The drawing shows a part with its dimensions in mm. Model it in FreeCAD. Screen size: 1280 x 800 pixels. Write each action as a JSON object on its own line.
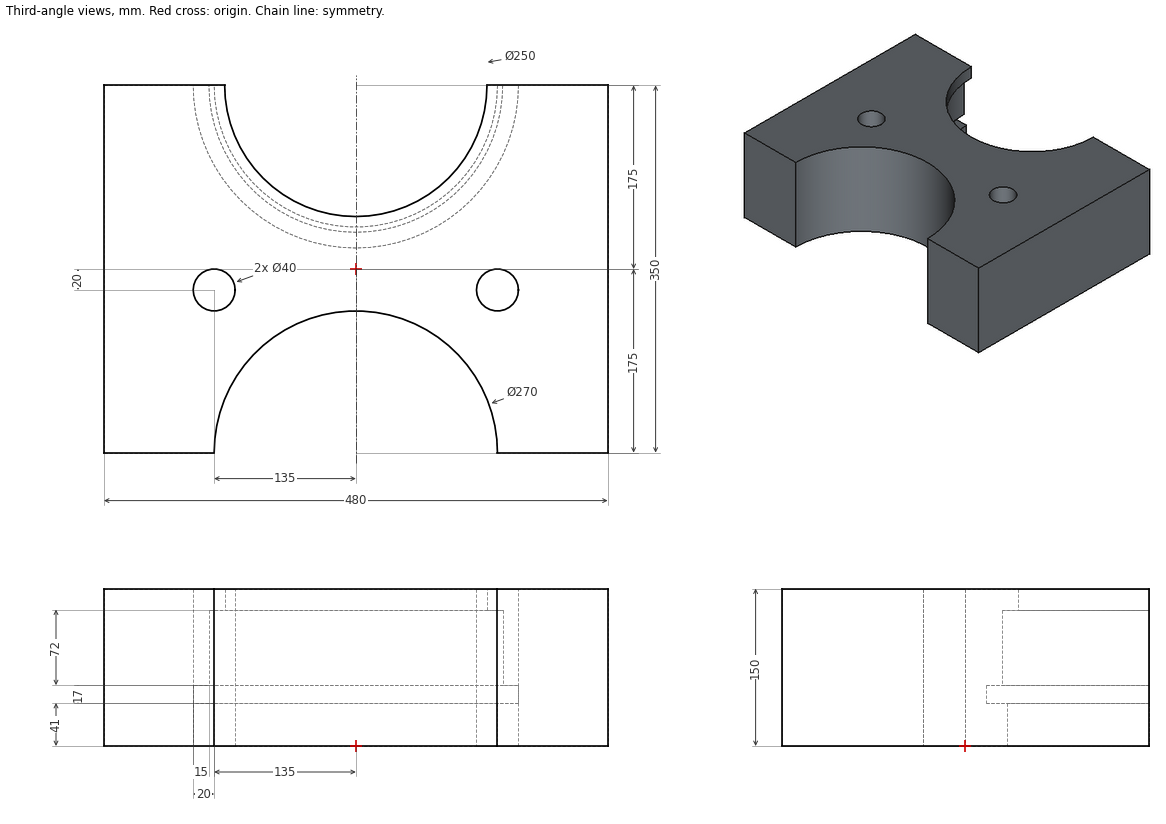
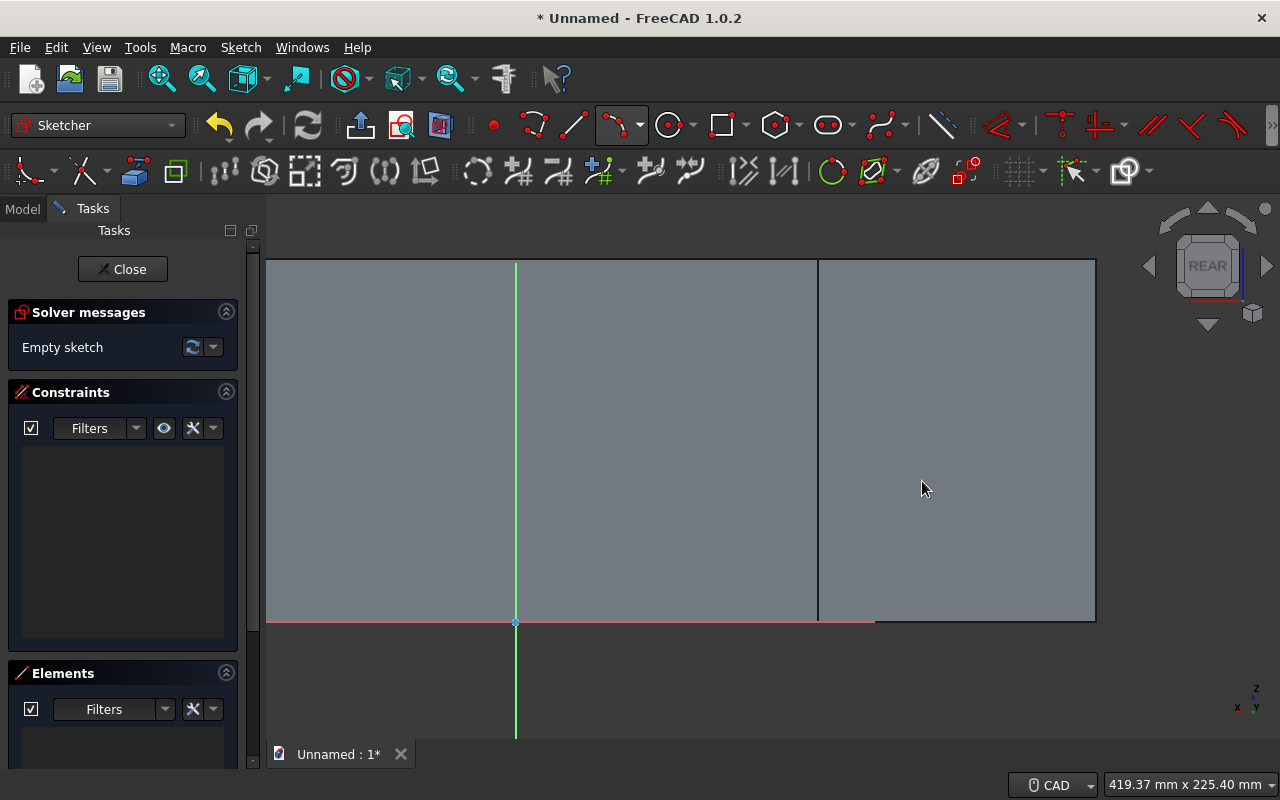
{"action": "left_click", "coordinate": [534, 126]}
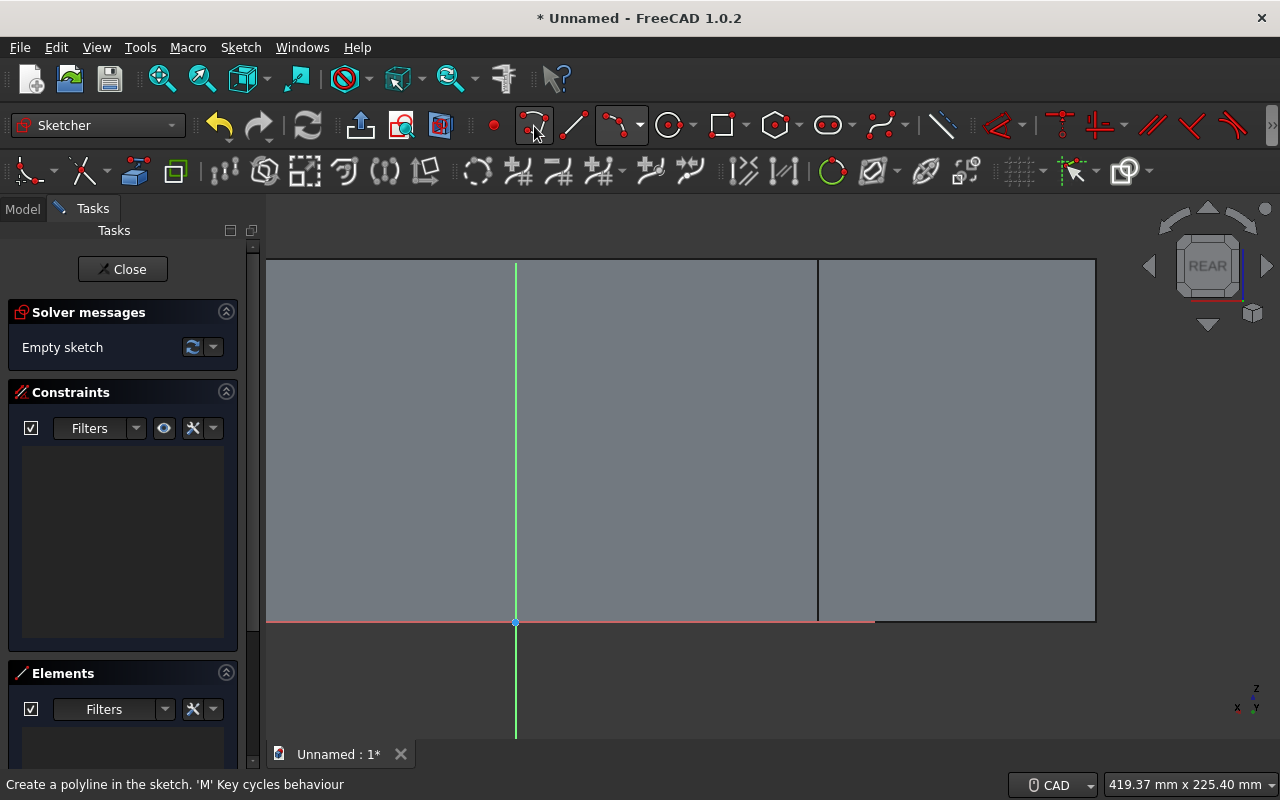
{"action": "left_click", "coordinate": [516, 622]}
{"action": "left_click", "coordinate": [842, 613]}
{"action": "left_click", "coordinate": [842, 523]}
{"action": "left_click", "coordinate": [891, 523]}
{"action": "left_click", "coordinate": [891, 482]}
{"action": "left_click", "coordinate": [854, 482]}
{"action": "left_click", "coordinate": [854, 308]}
{"action": "left_click", "coordinate": [525, 308]}
{"action": "left_click", "coordinate": [516, 622]}
{"action": "key", "text": "Escape"}
{"action": "key", "text": "Escape"}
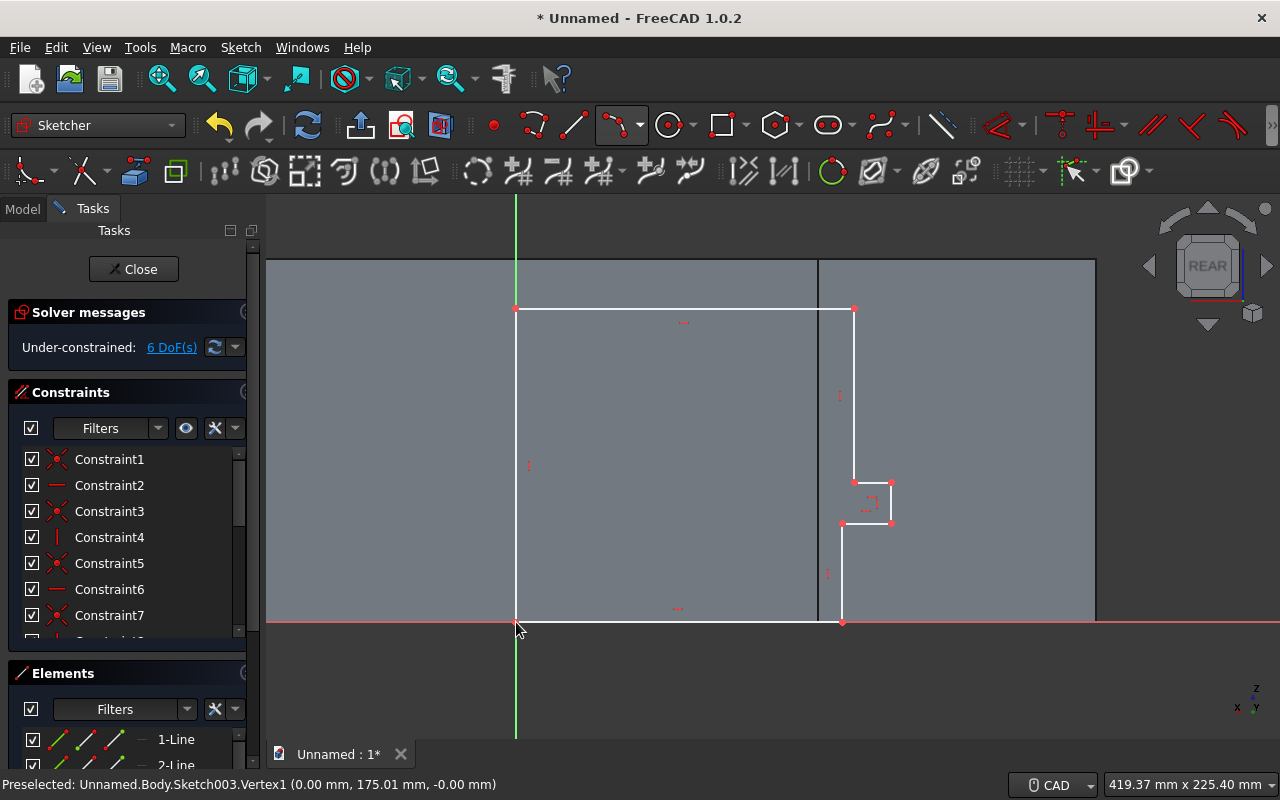
{"action": "key", "text": "d"}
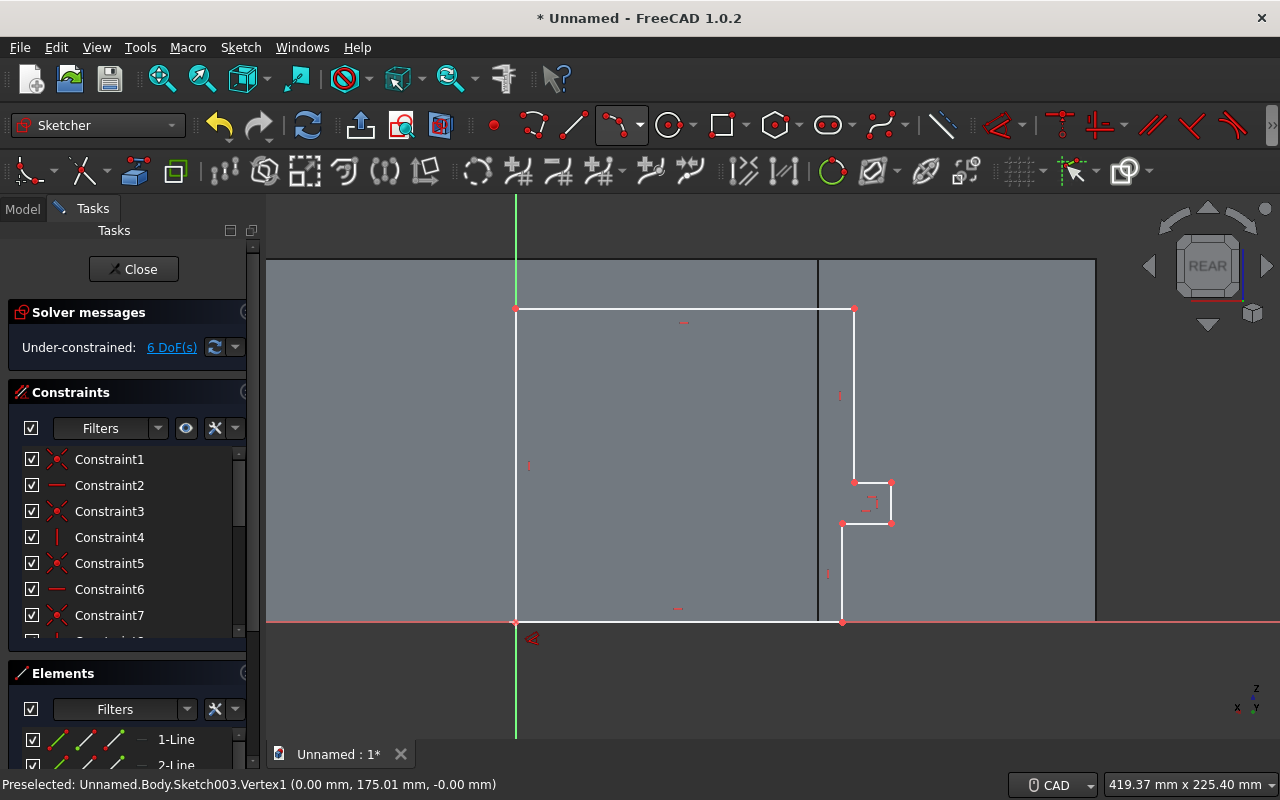
{"action": "left_click", "coordinate": [842, 593]}
{"action": "left_click", "coordinate": [876, 573]}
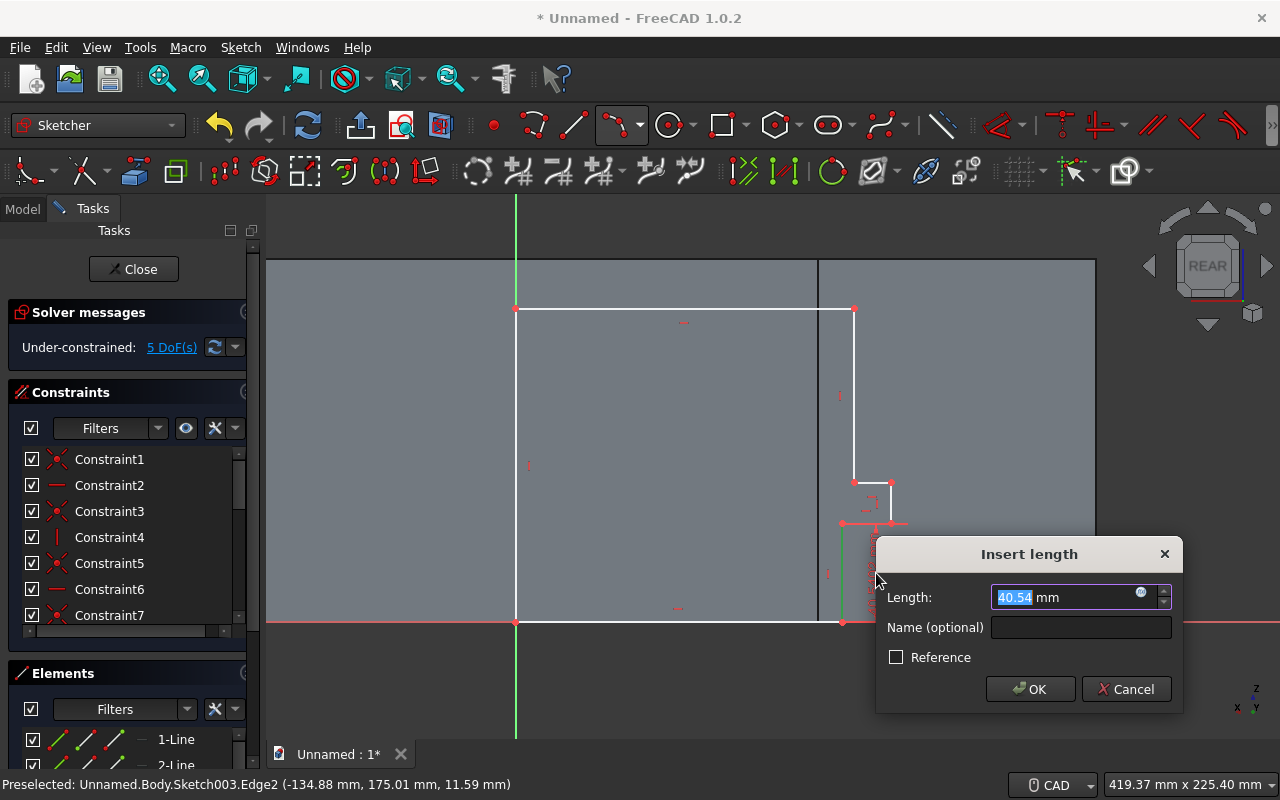
{"action": "type", "text": "41"}
{"action": "key", "text": "Return"}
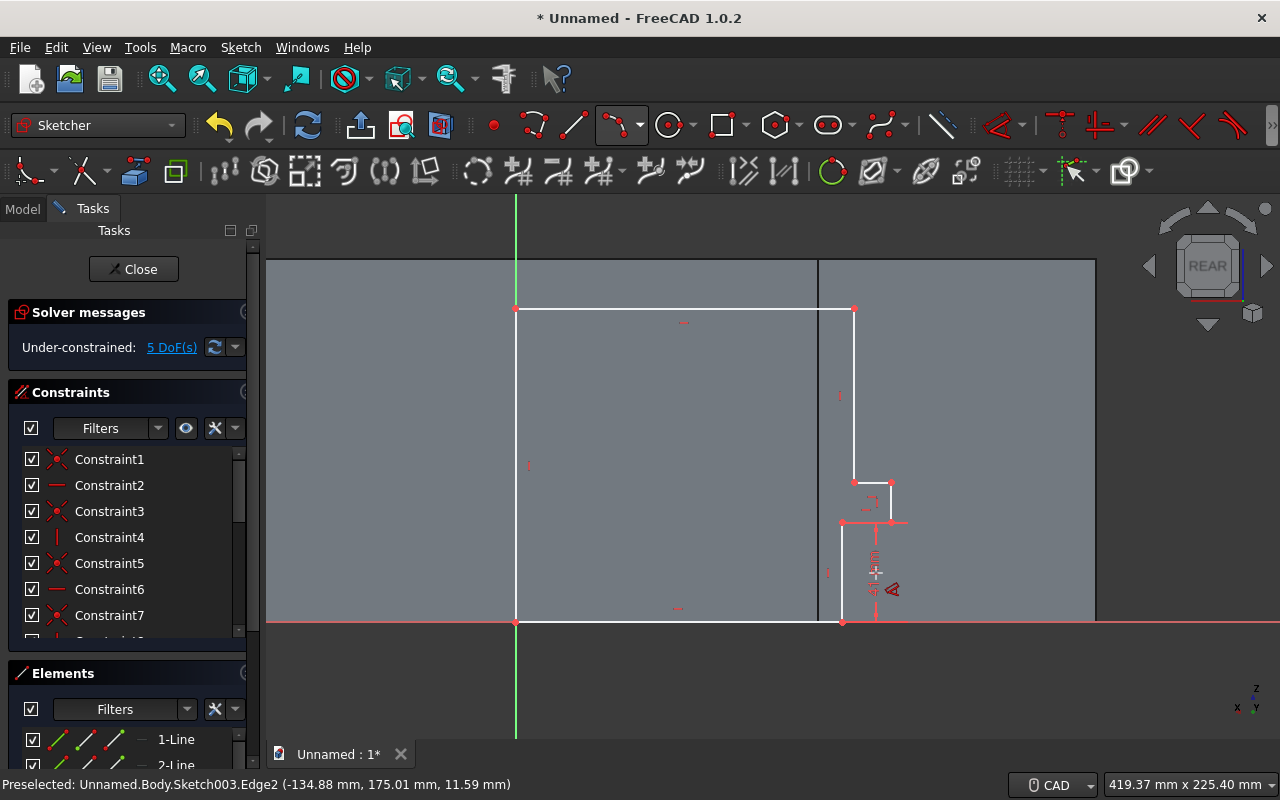
{"action": "left_click", "coordinate": [857, 523]}
{"action": "left_click", "coordinate": [878, 465]}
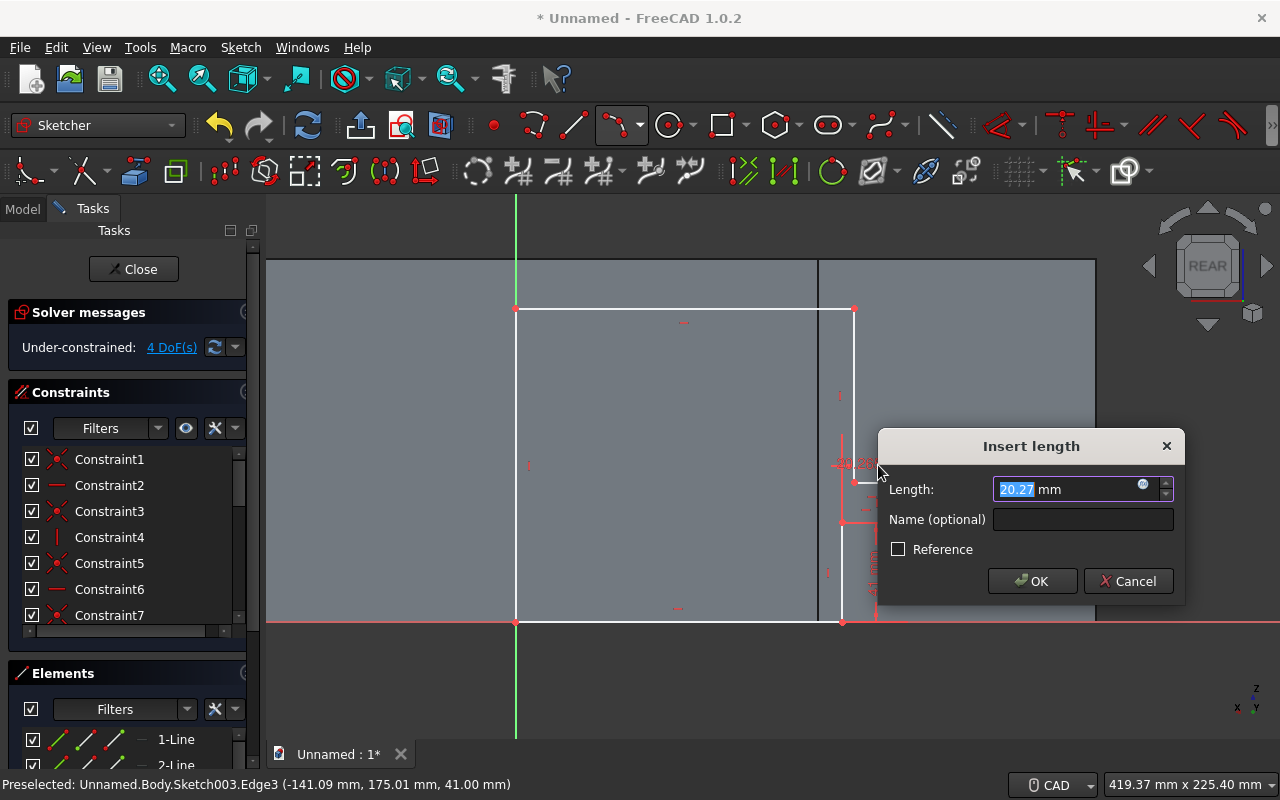
{"action": "type", "text": "20"}
{"action": "key", "text": "Return"}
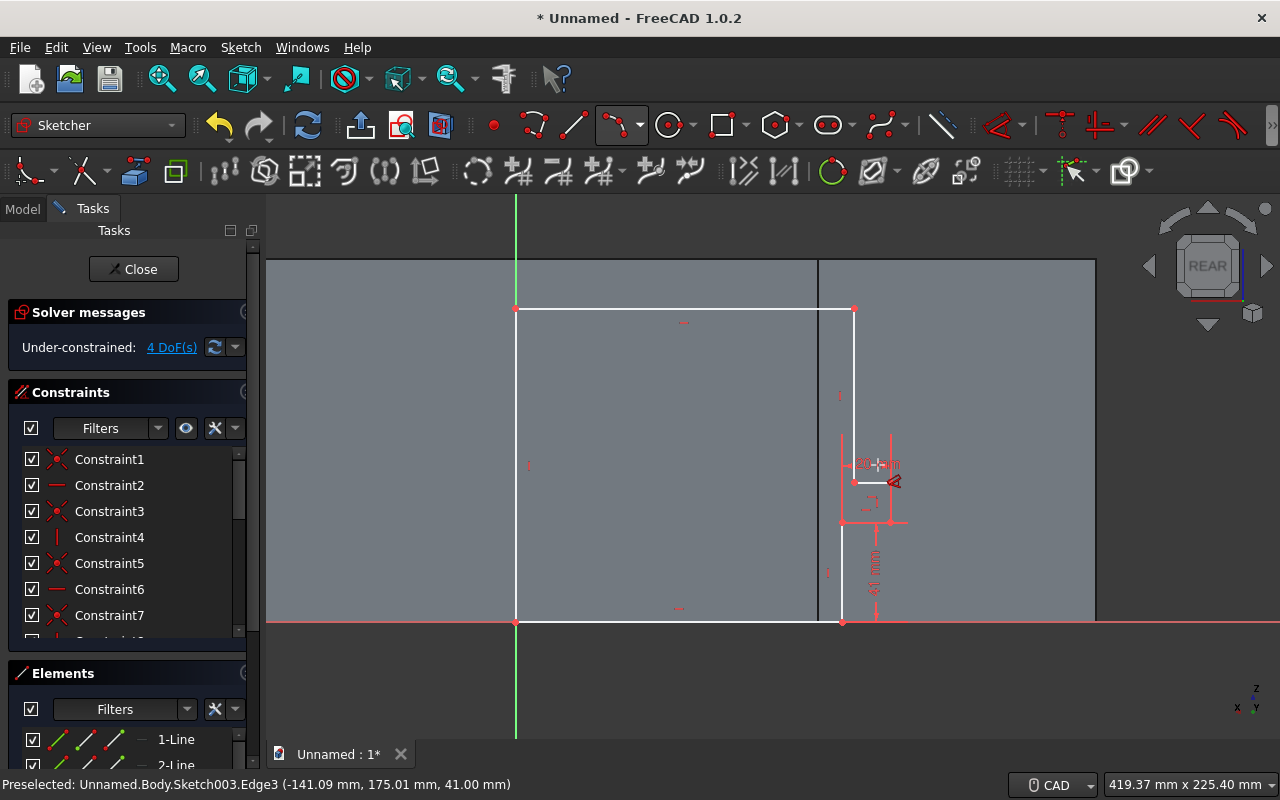
{"action": "left_click", "coordinate": [891, 511]}
{"action": "left_click", "coordinate": [925, 503]}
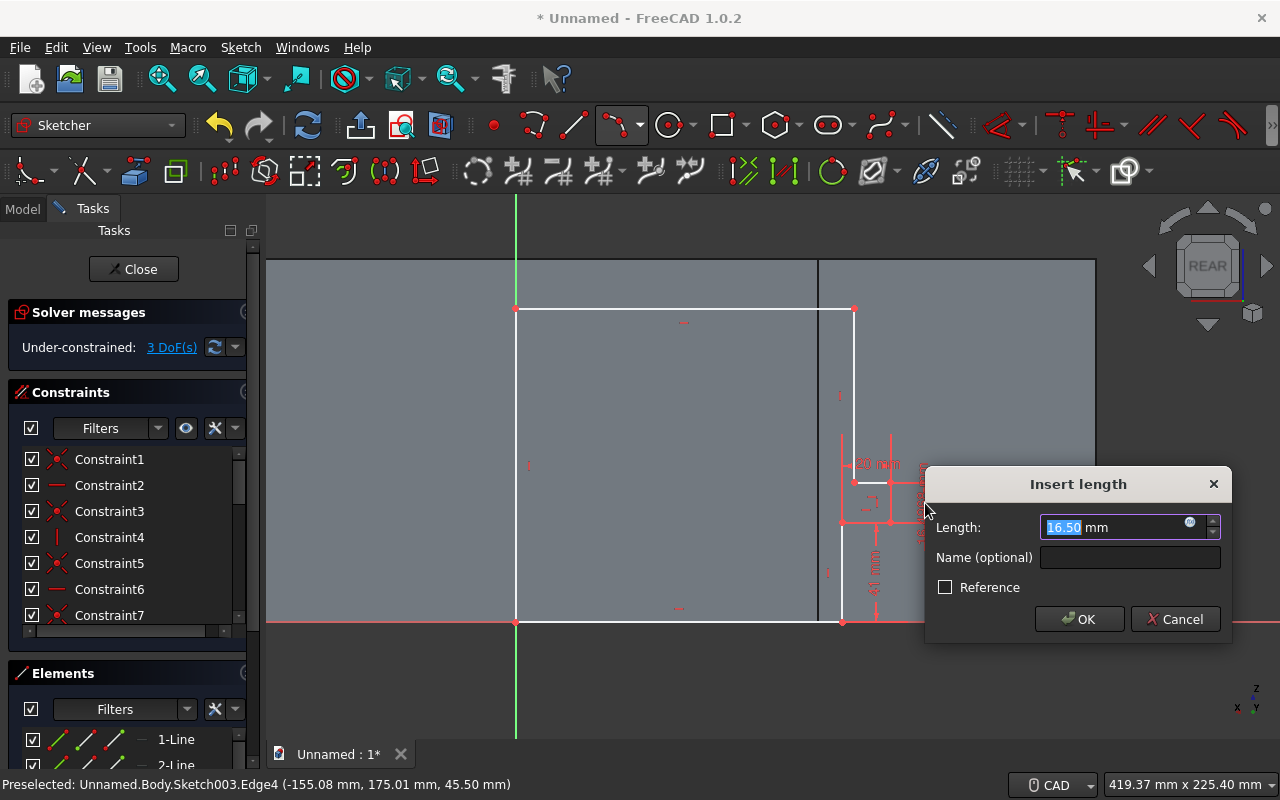
{"action": "type", "text": "17"}
{"action": "key", "text": "Return"}